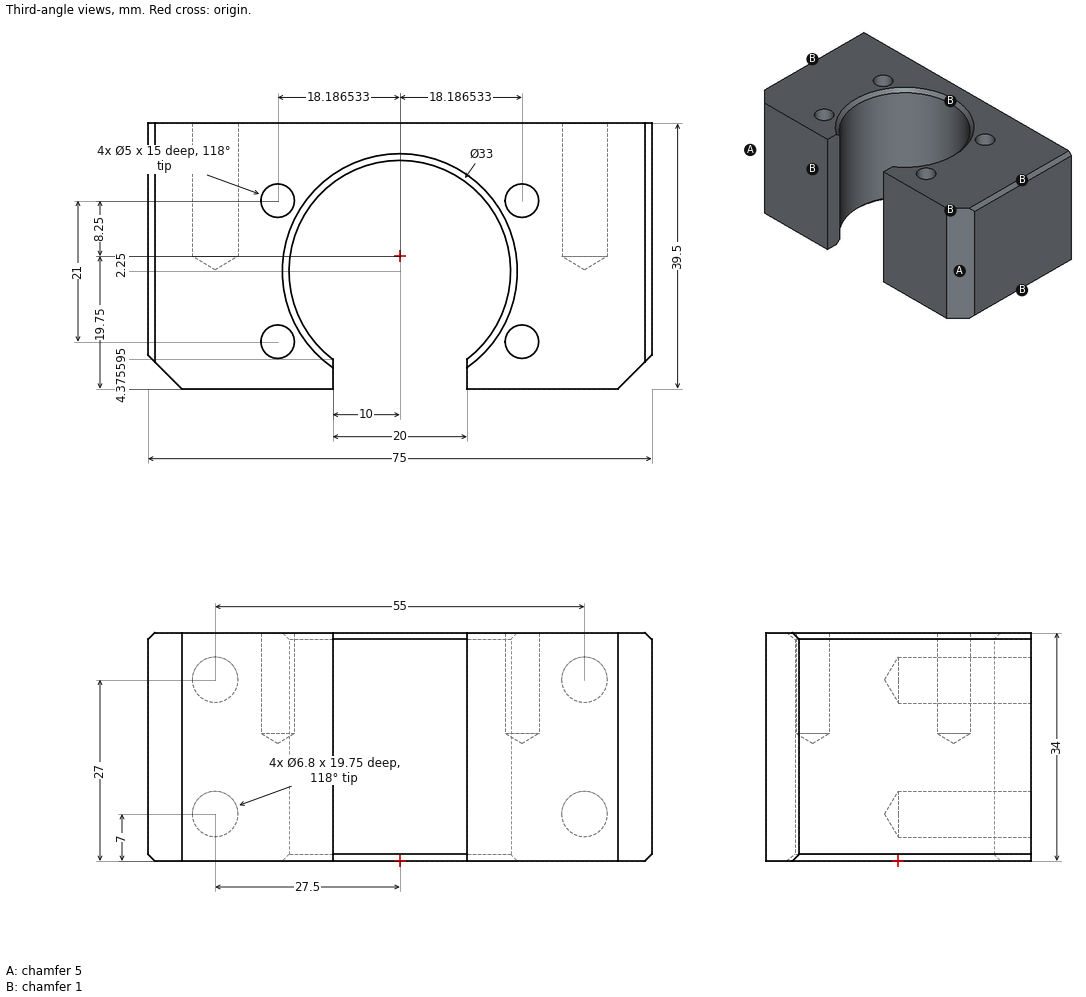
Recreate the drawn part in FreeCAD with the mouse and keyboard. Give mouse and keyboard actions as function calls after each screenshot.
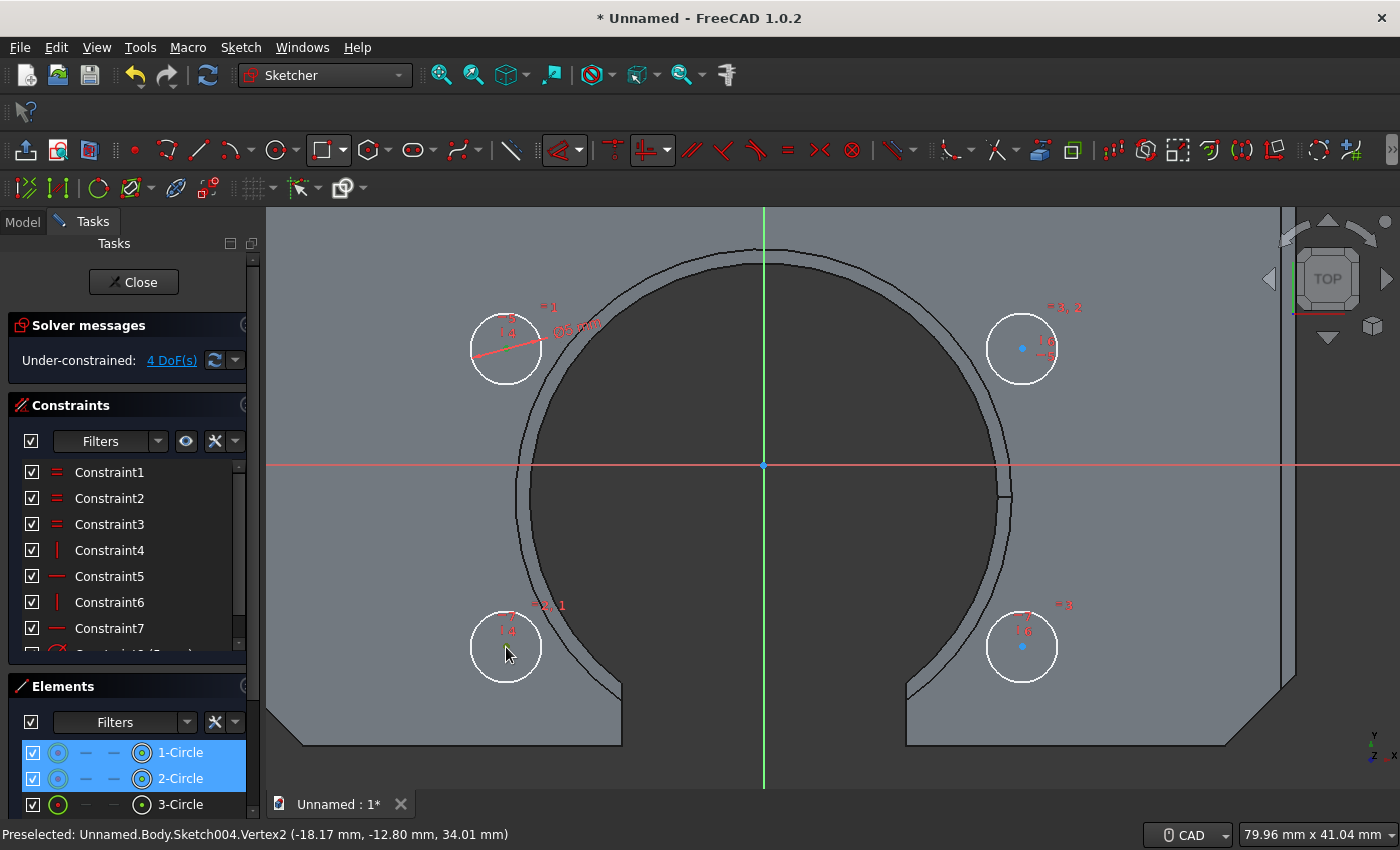
key(i)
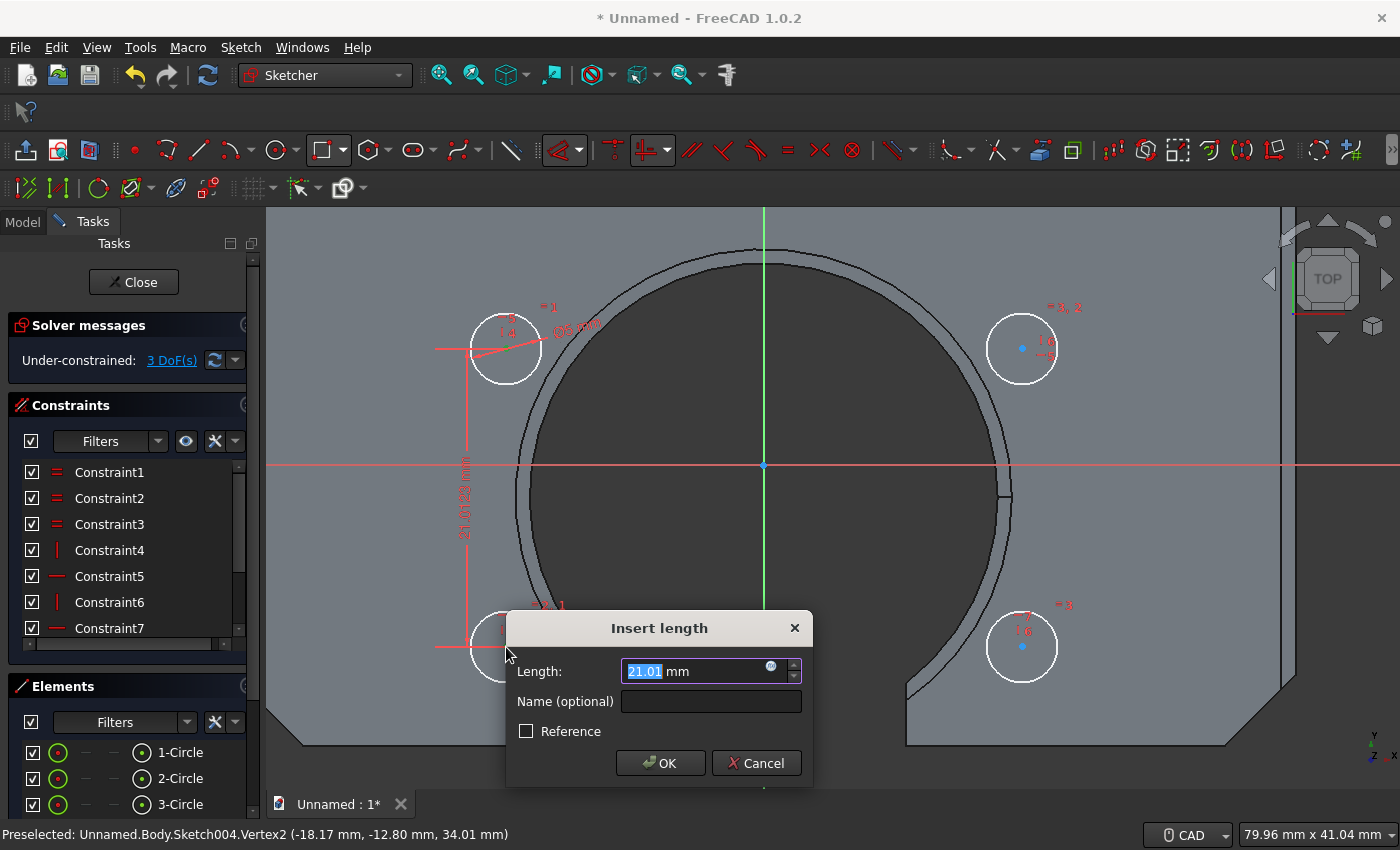
text(21)
key(Return)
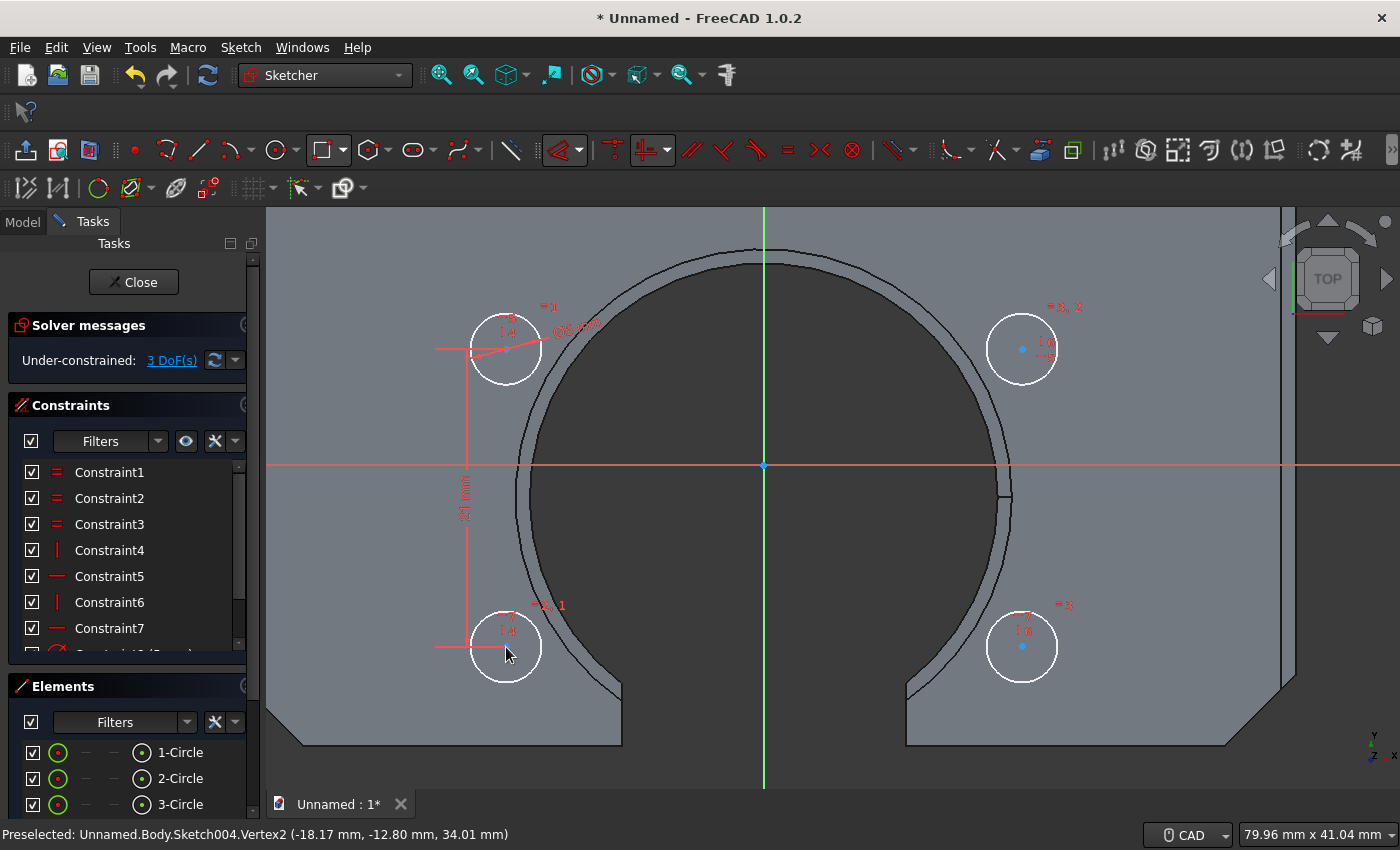
click(506, 349)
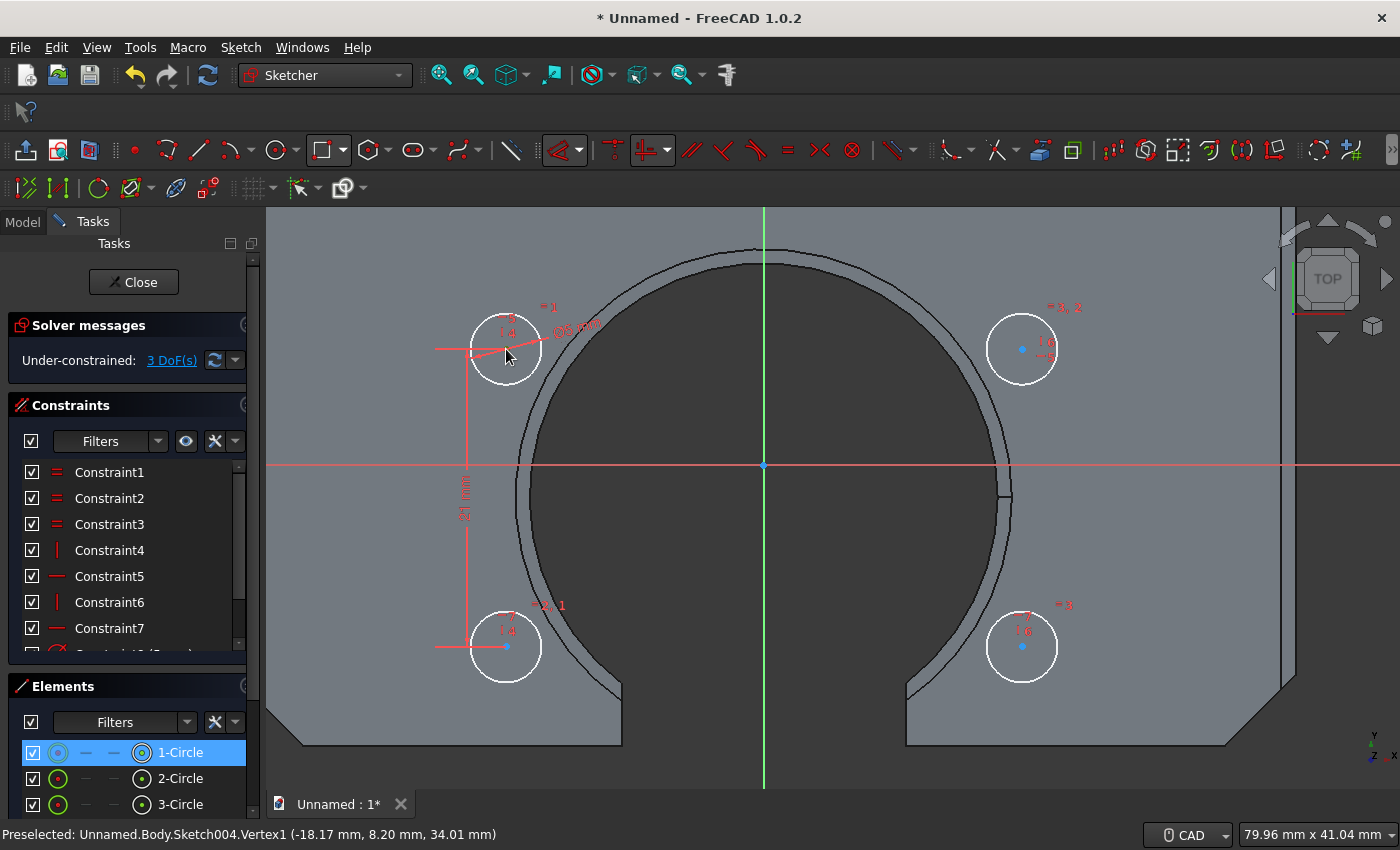
key(i)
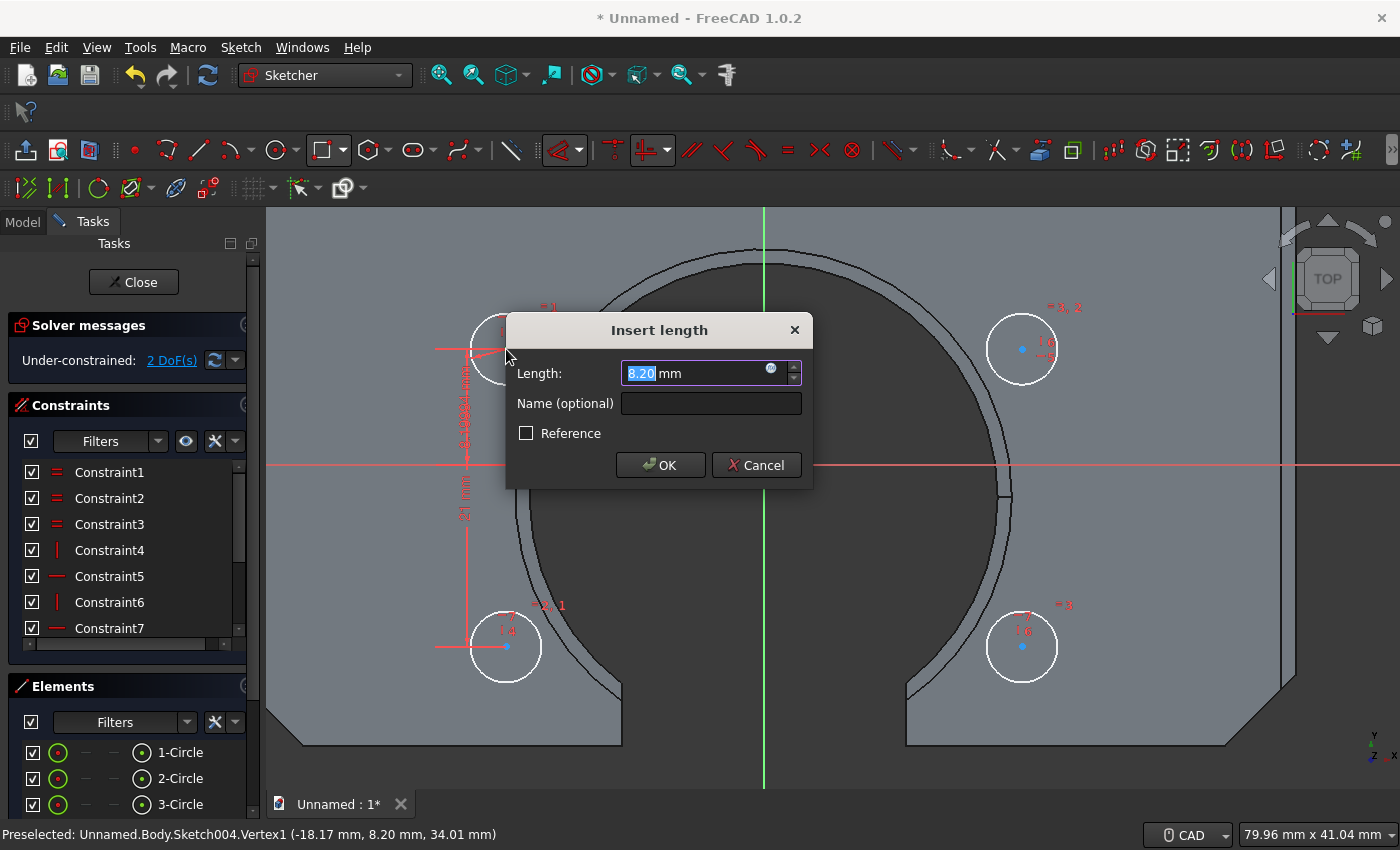
text(8.25)
key(Return)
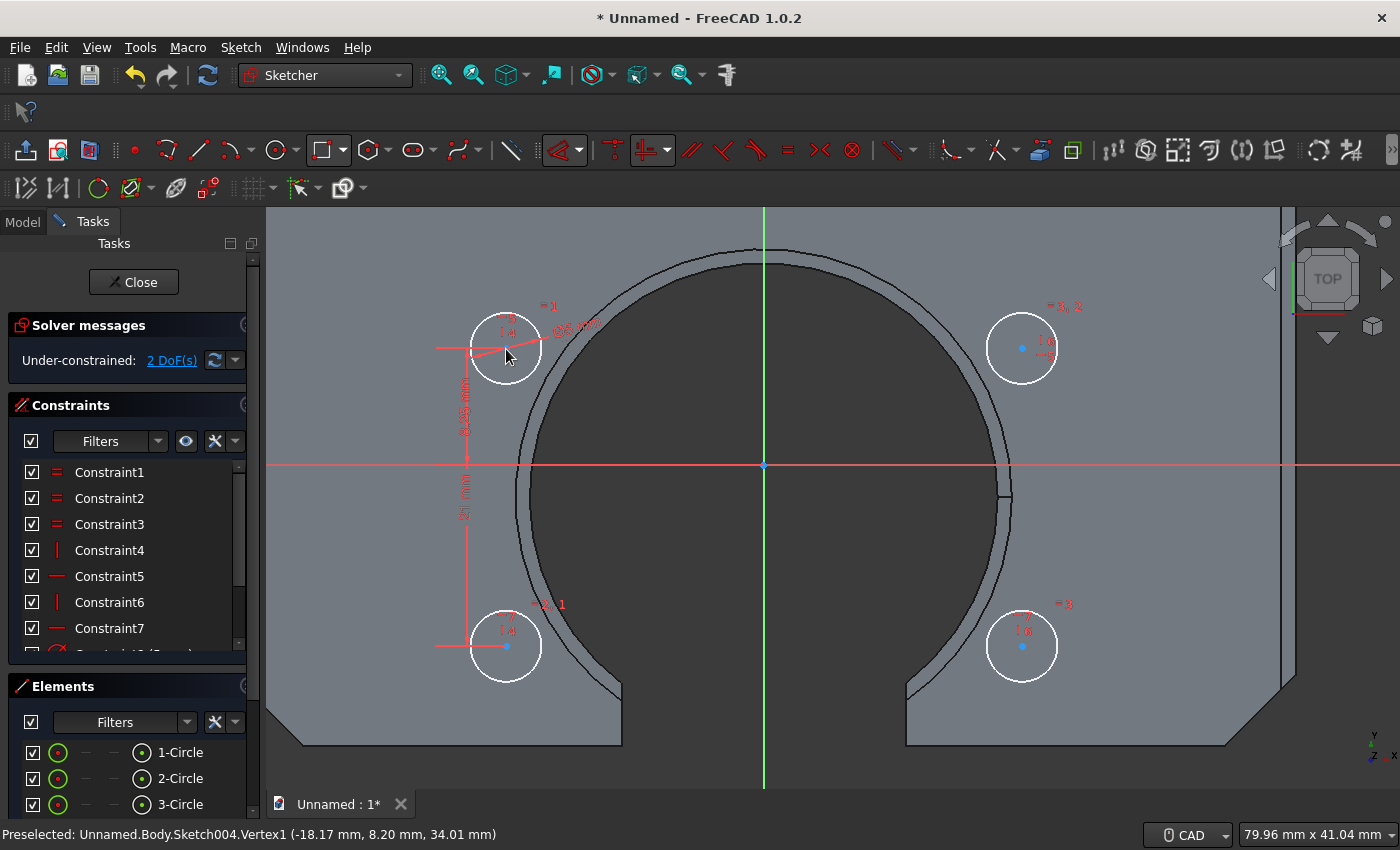
click(506, 348)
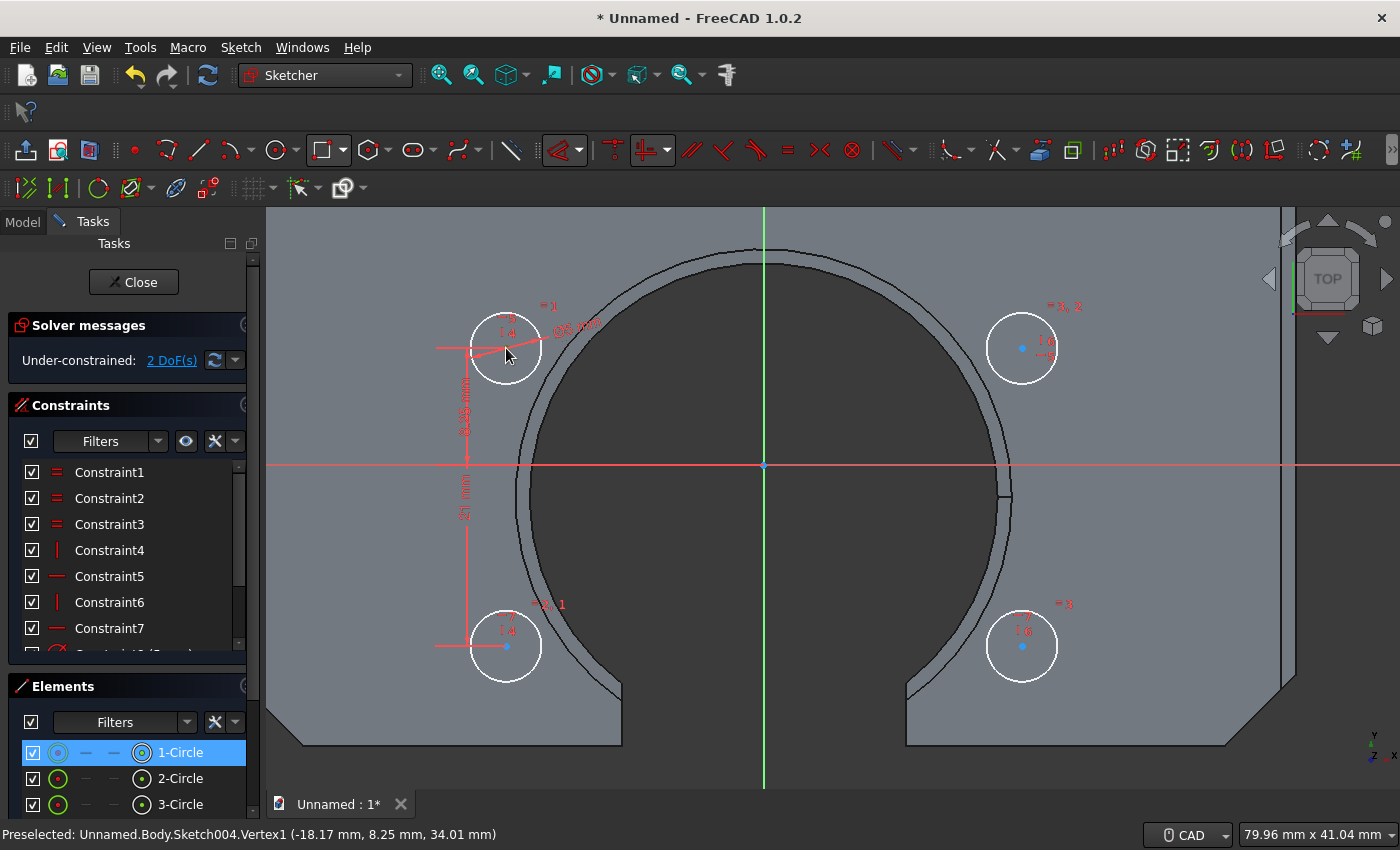
click(582, 150)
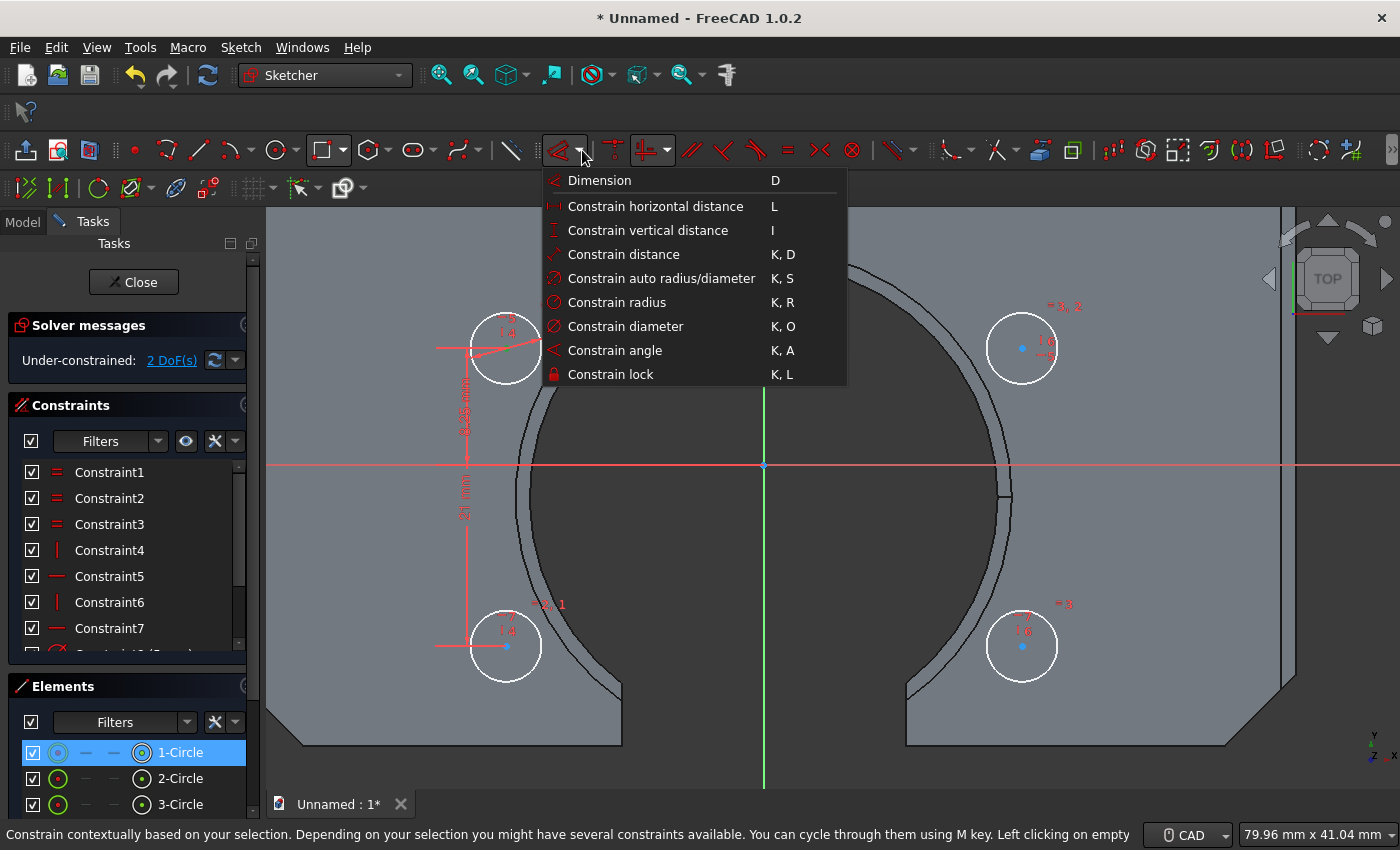
click(695, 206)